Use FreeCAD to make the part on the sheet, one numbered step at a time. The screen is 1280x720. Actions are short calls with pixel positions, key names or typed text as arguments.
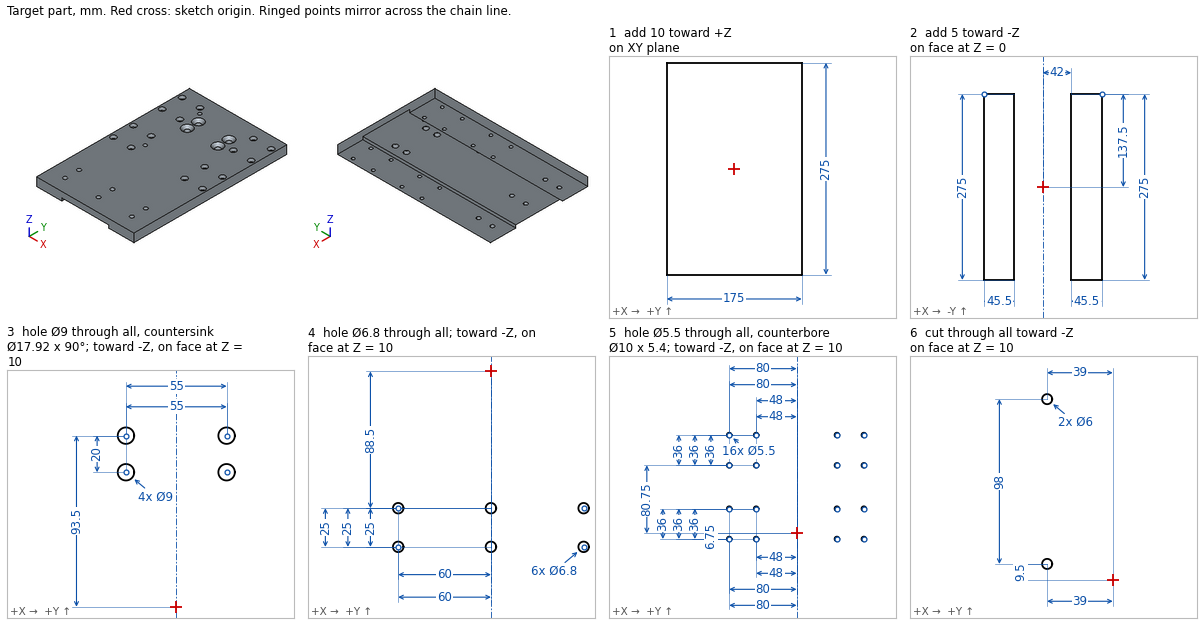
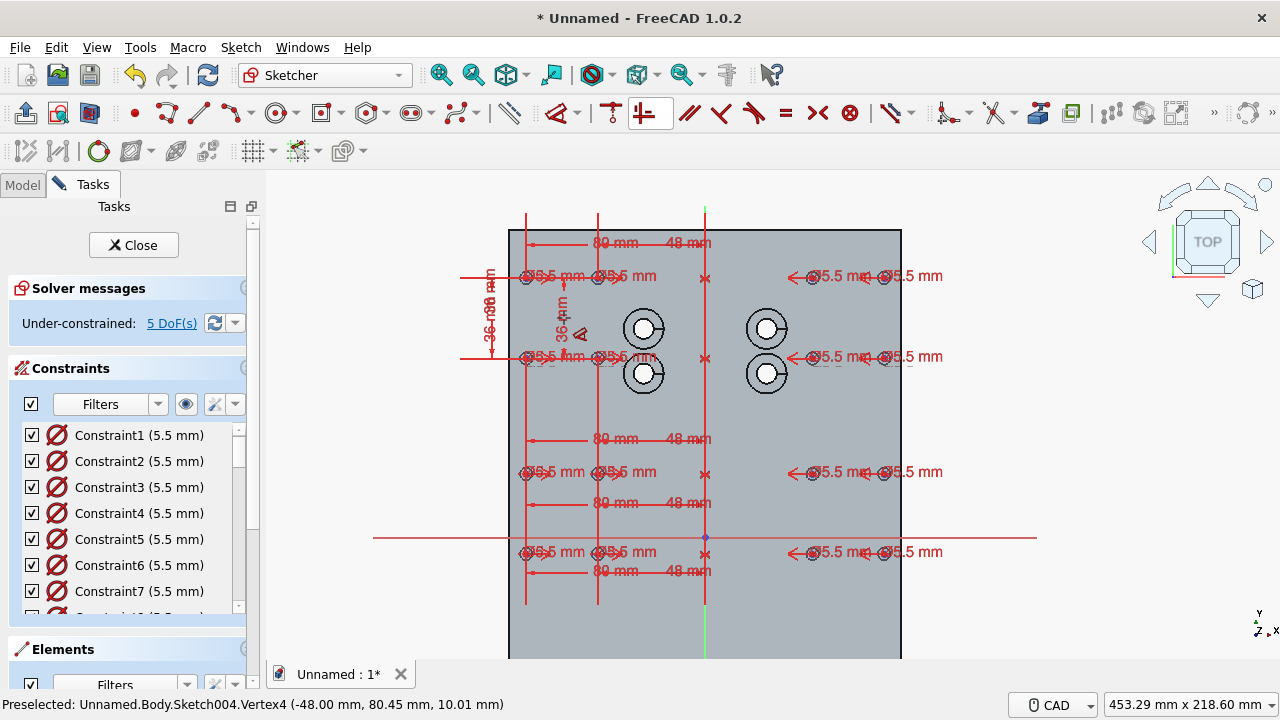
click(526, 474)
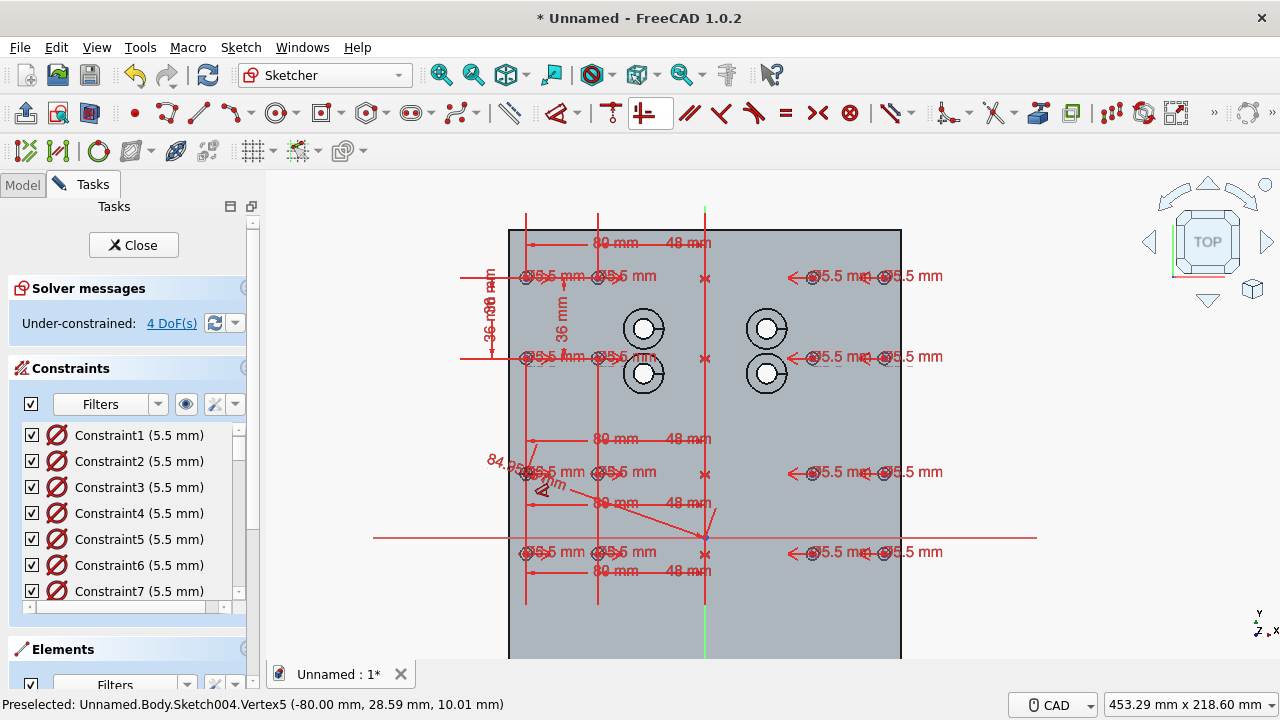
click(526, 554)
click(492, 514)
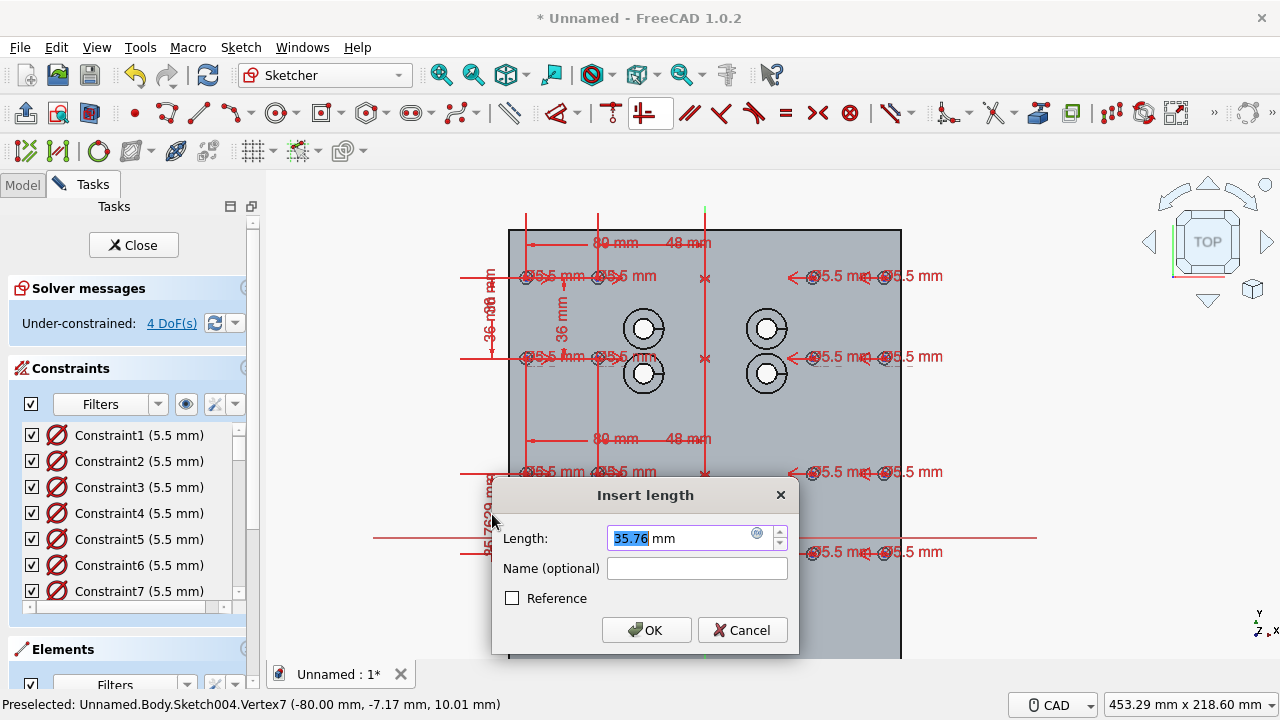
text(36)
key(Return)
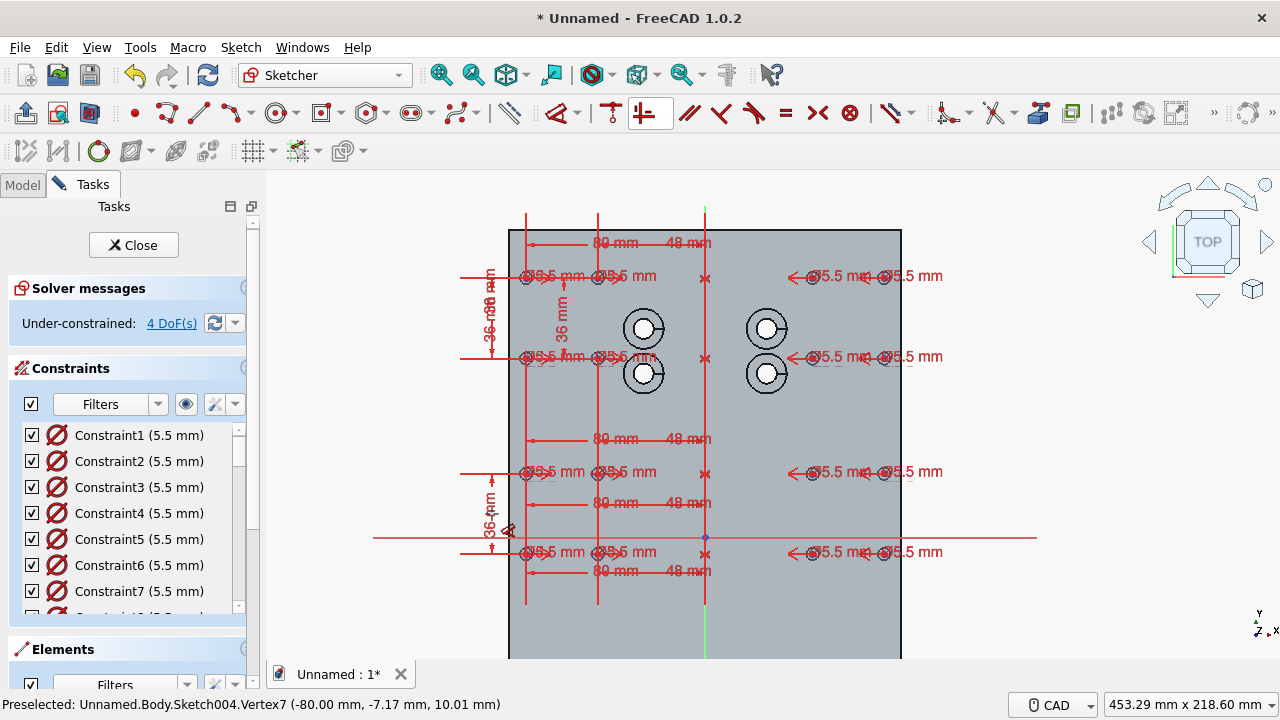
click(598, 474)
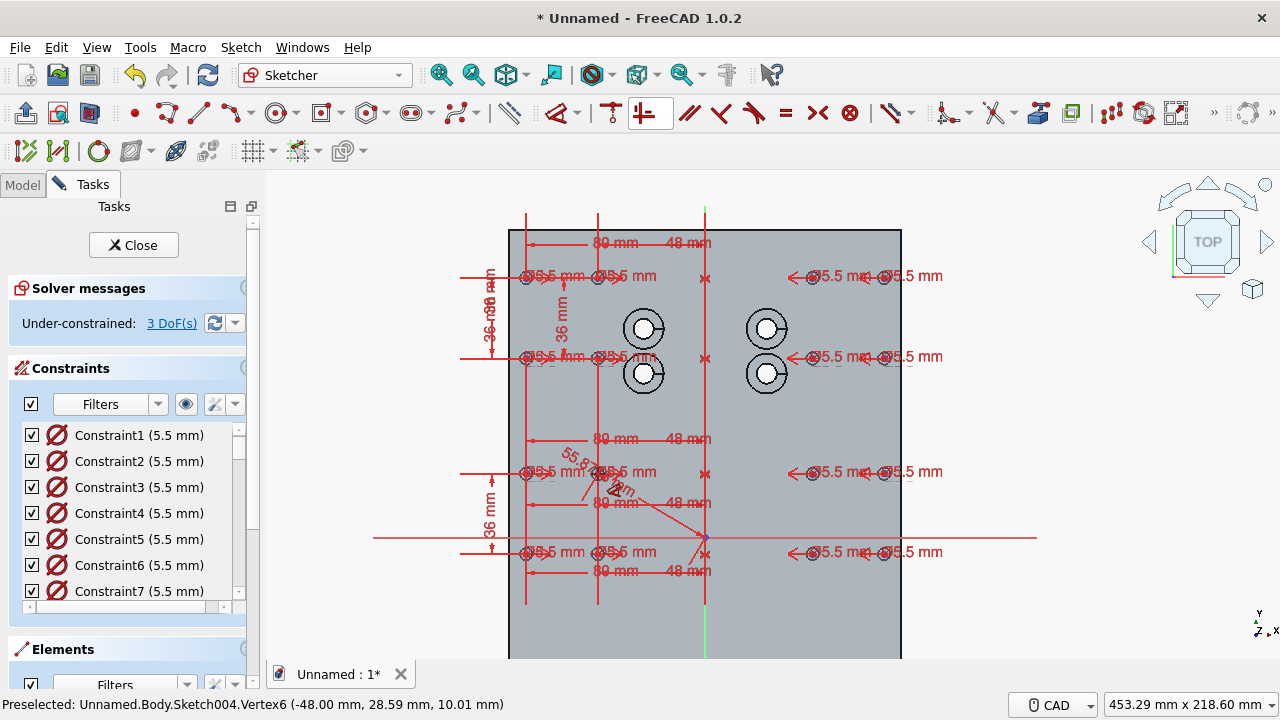
click(526, 554)
click(492, 486)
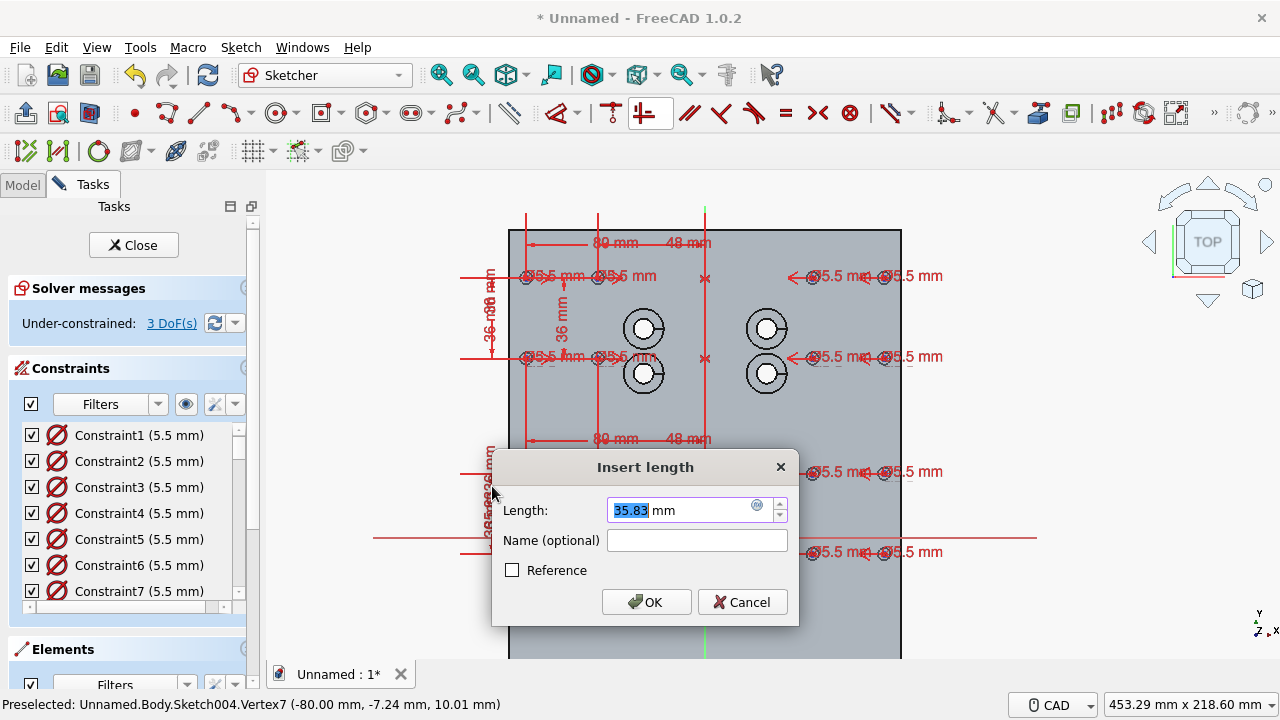
text(36)
key(Return)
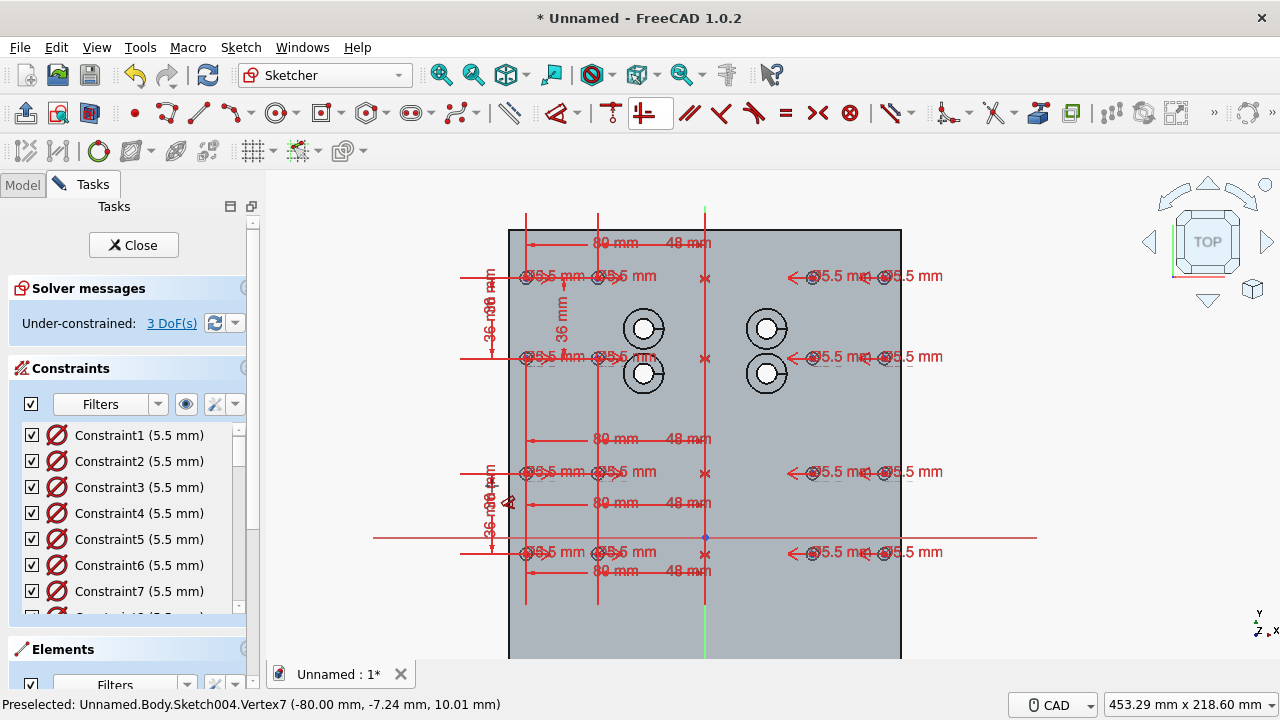
click(598, 474)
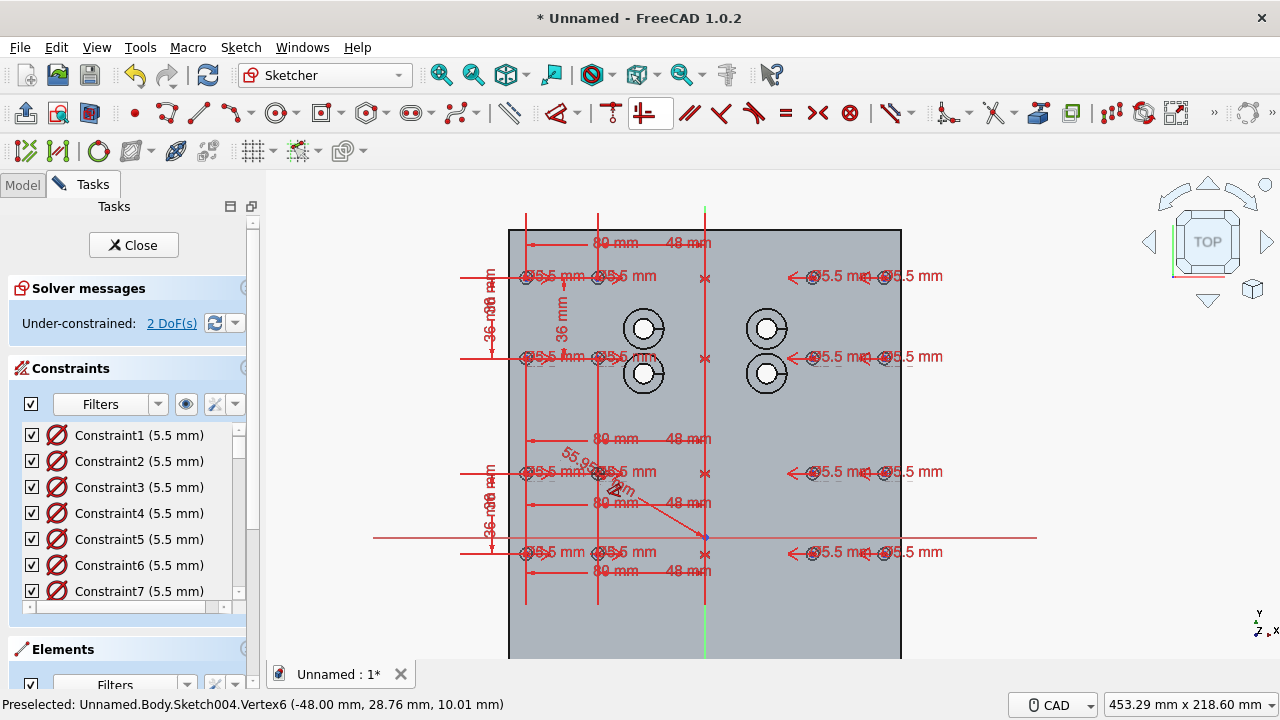
click(598, 554)
click(418, 514)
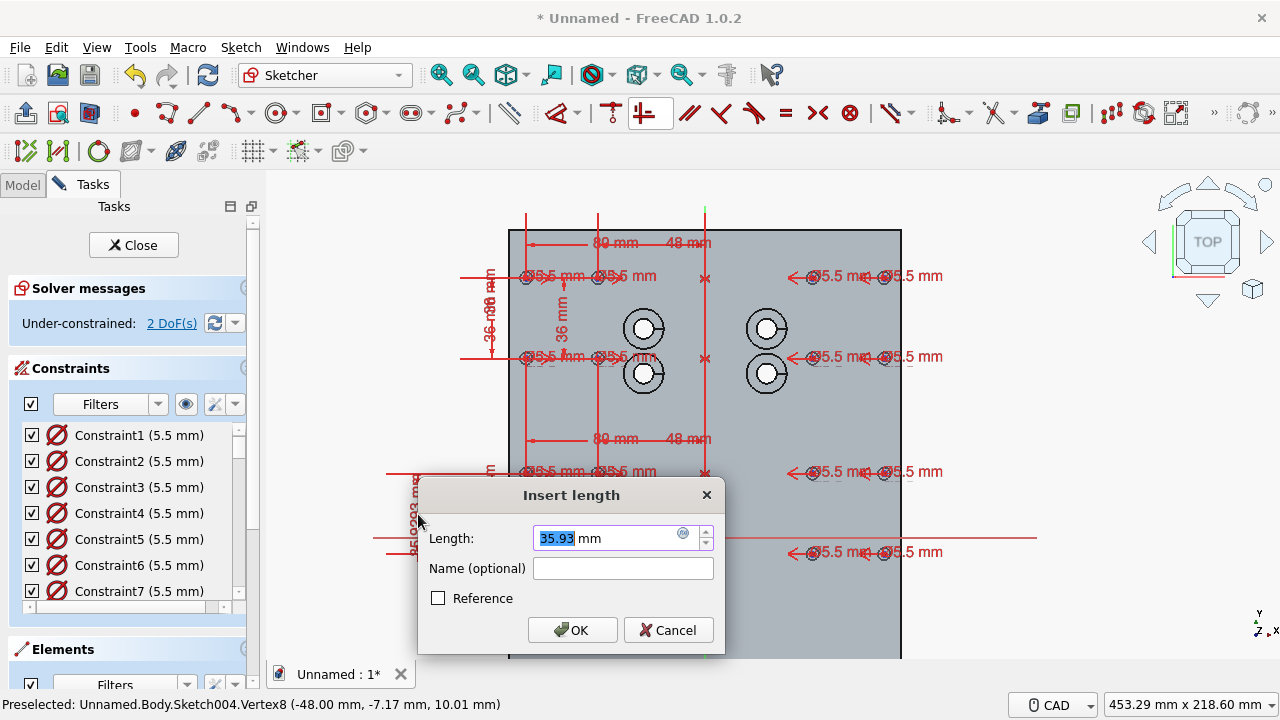
text(36)
key(Return)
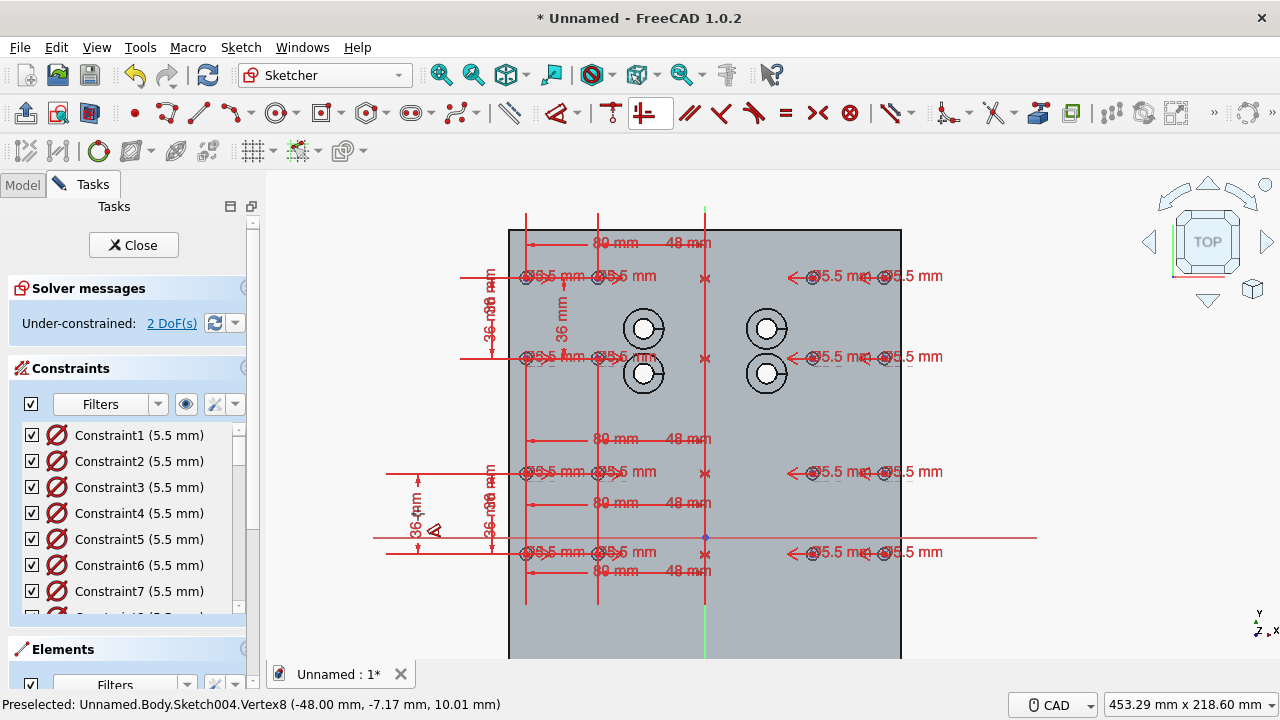
scroll(526, 554, up, 5)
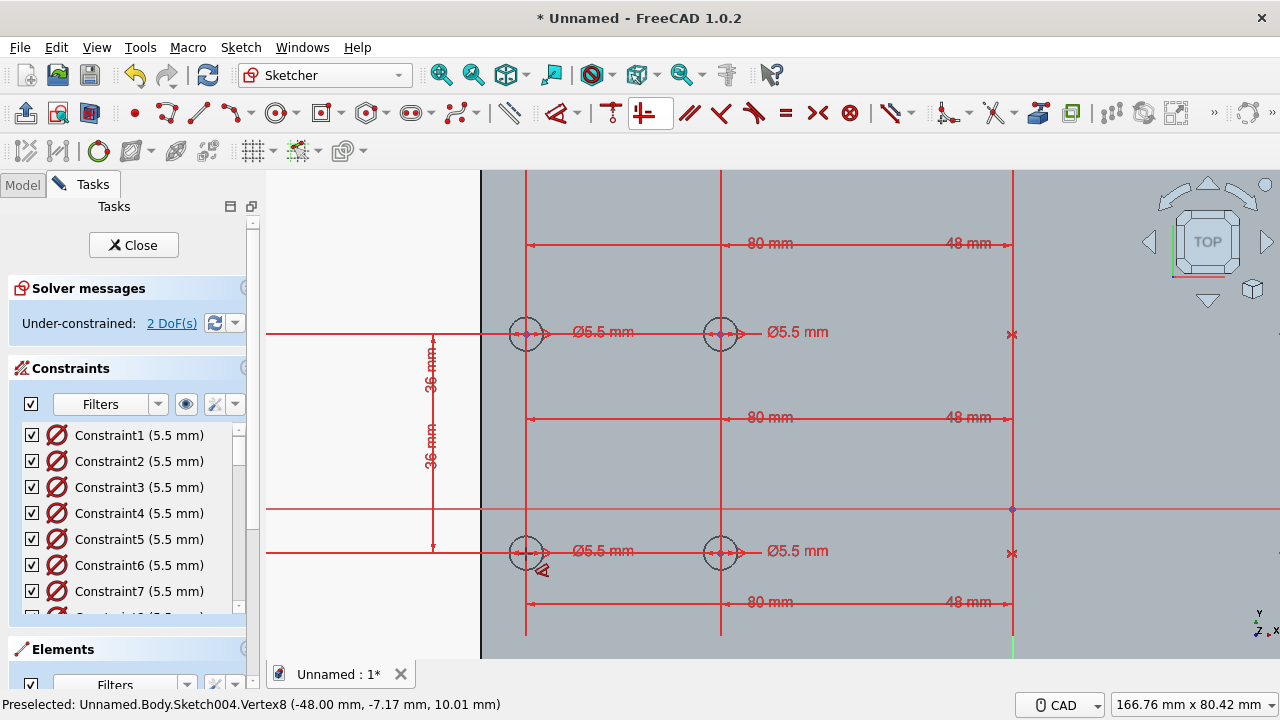
click(526, 553)
click(492, 531)